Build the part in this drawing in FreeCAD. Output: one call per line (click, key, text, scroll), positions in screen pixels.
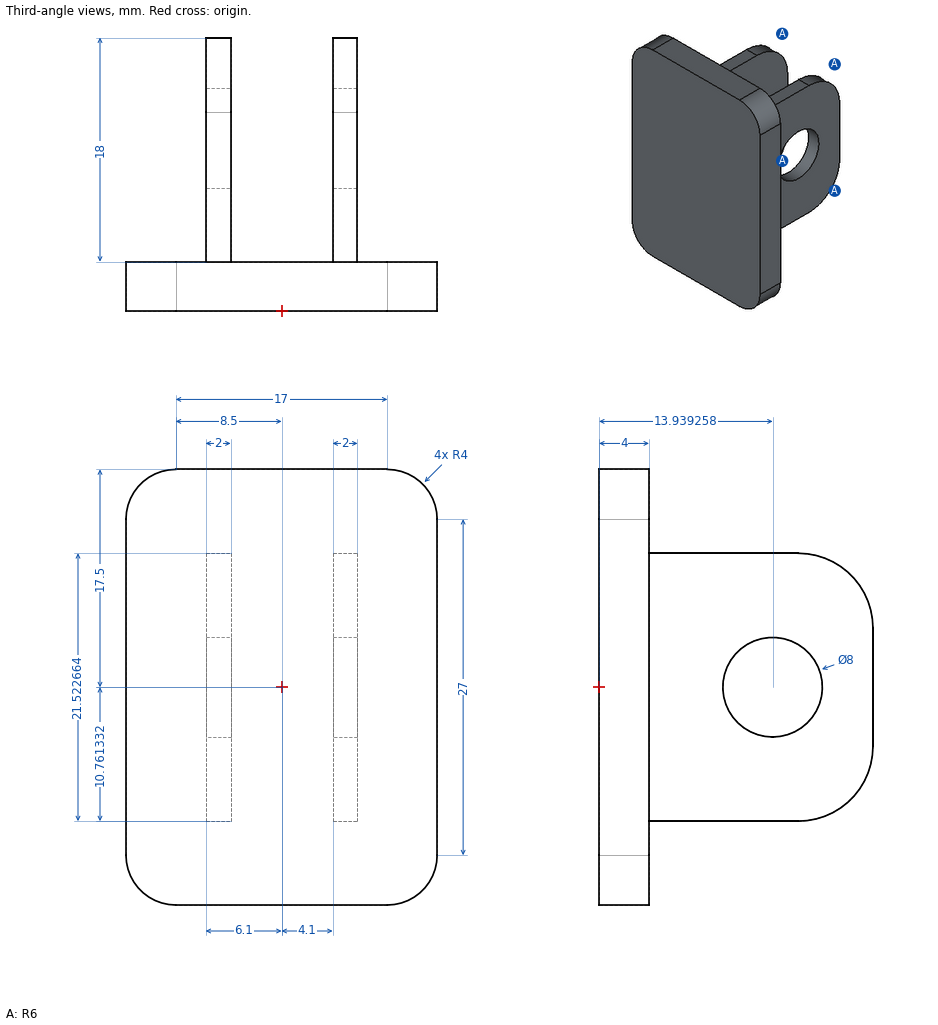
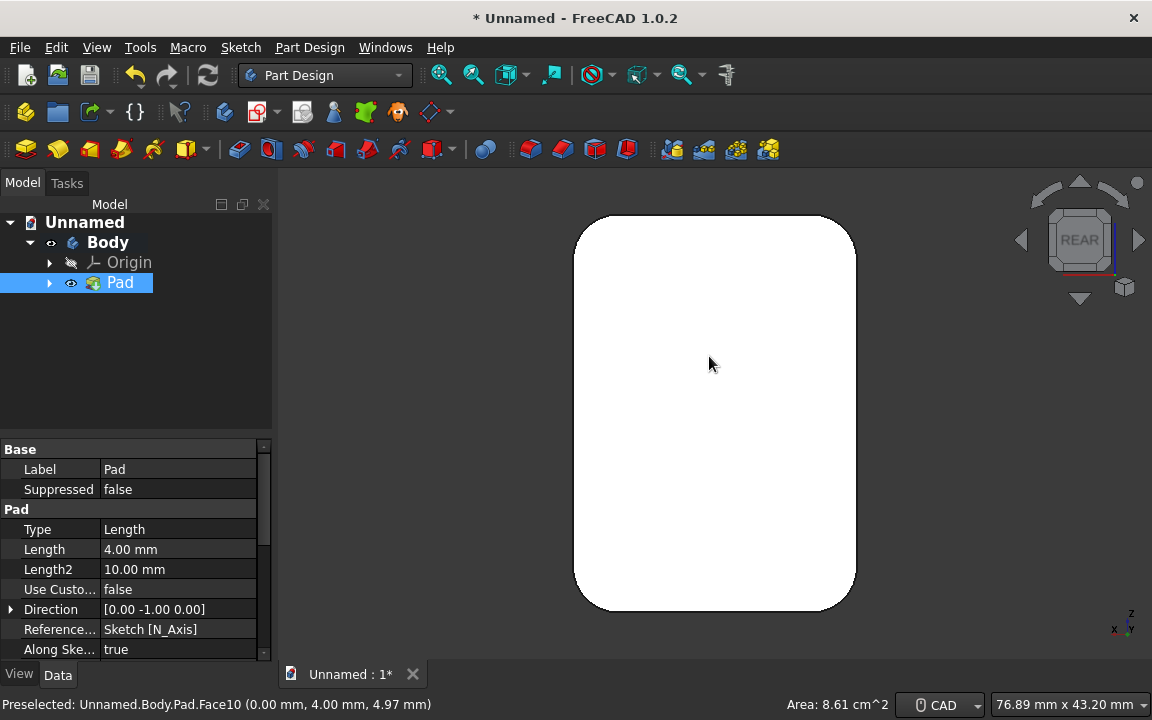
click(258, 112)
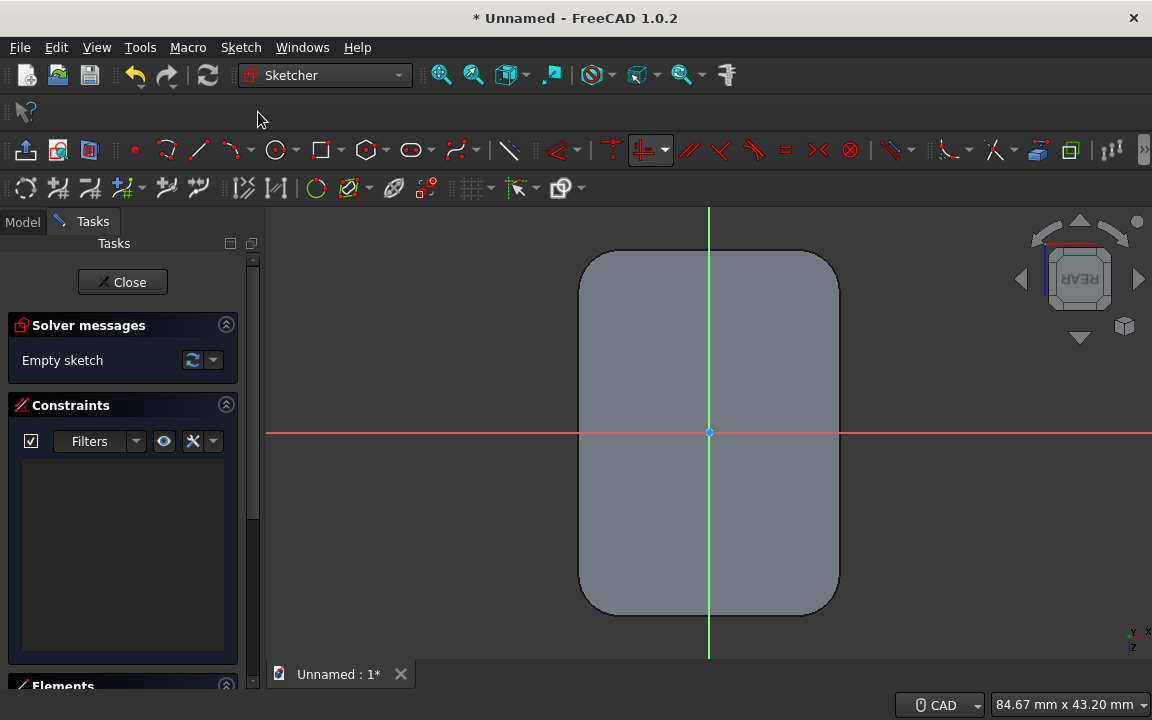
click(322, 150)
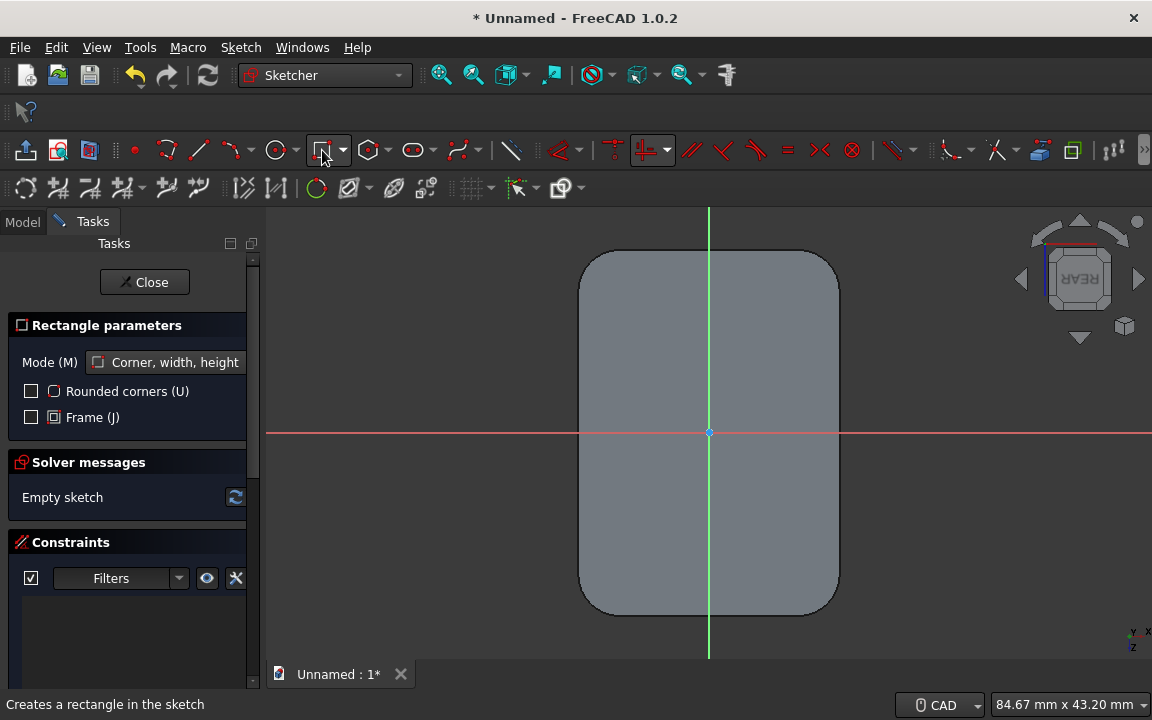
click(645, 320)
move(666, 546)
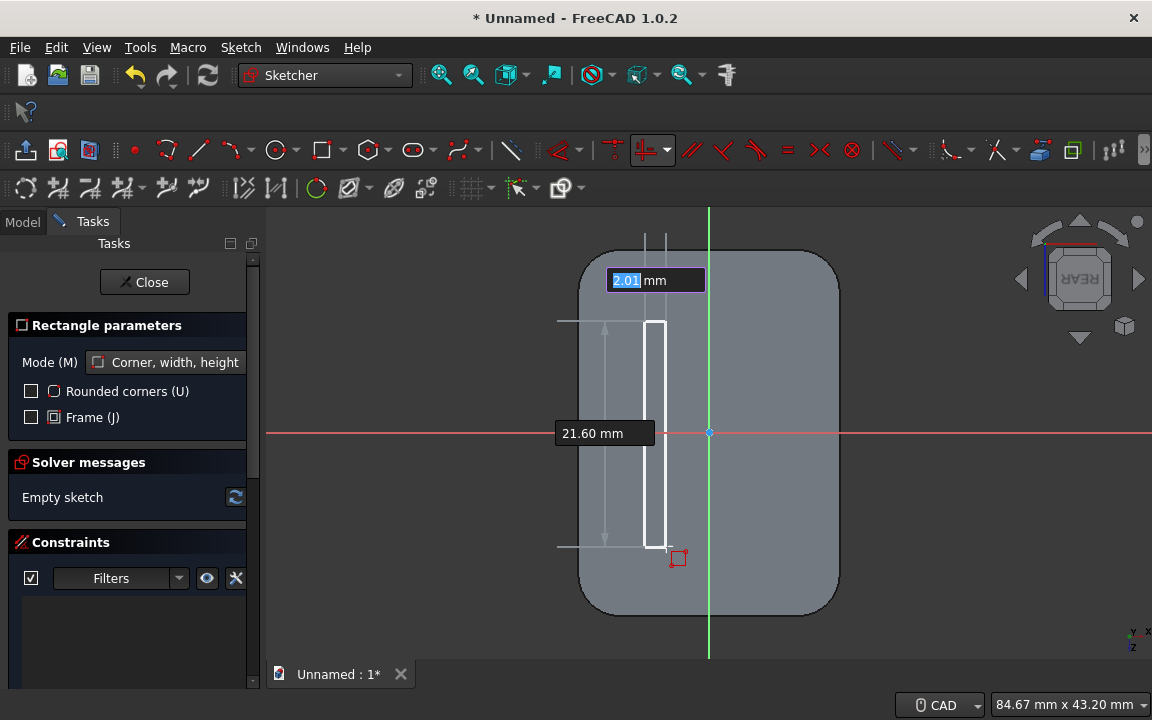
text(2)
key(Tab)
text(21.522664)
key(Return)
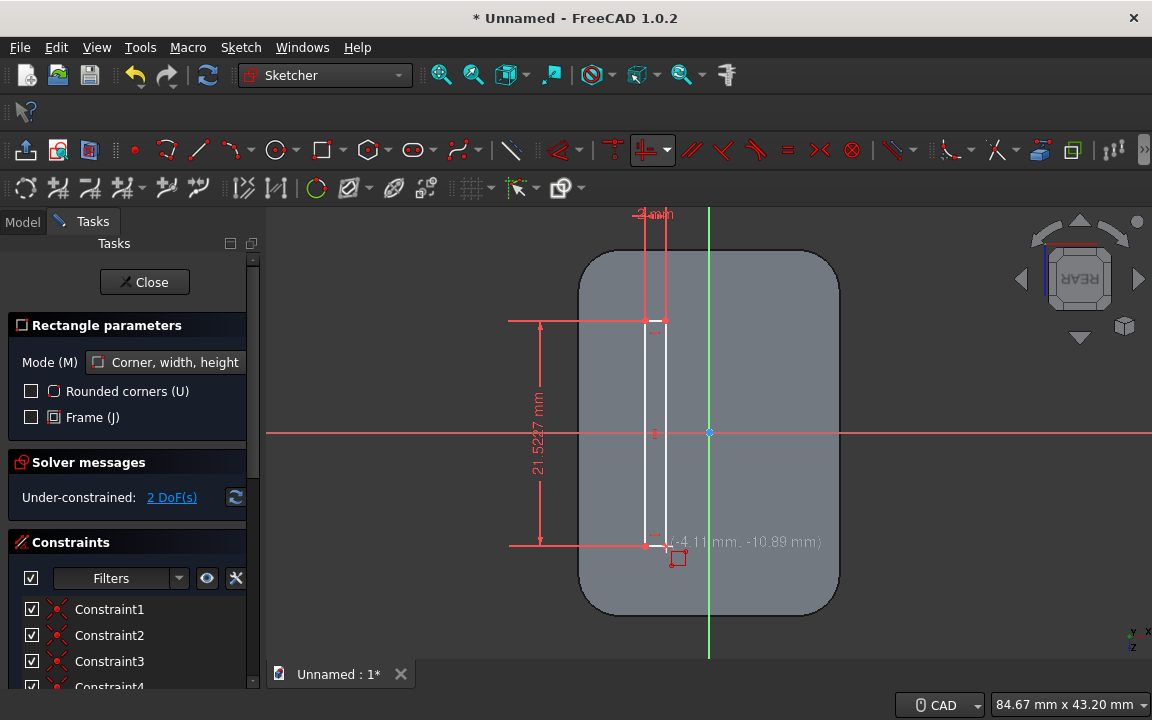
click(752, 320)
move(773, 546)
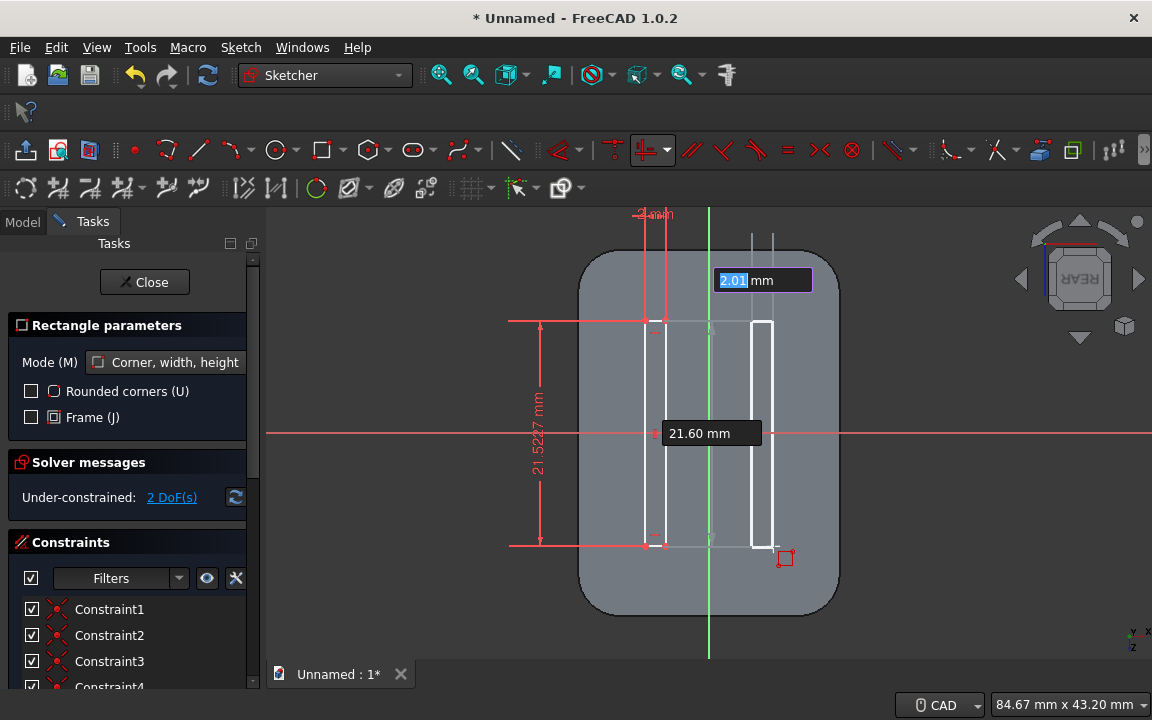
text(2)
key(Tab)
text(21.522664)
key(Return)
key(Escape)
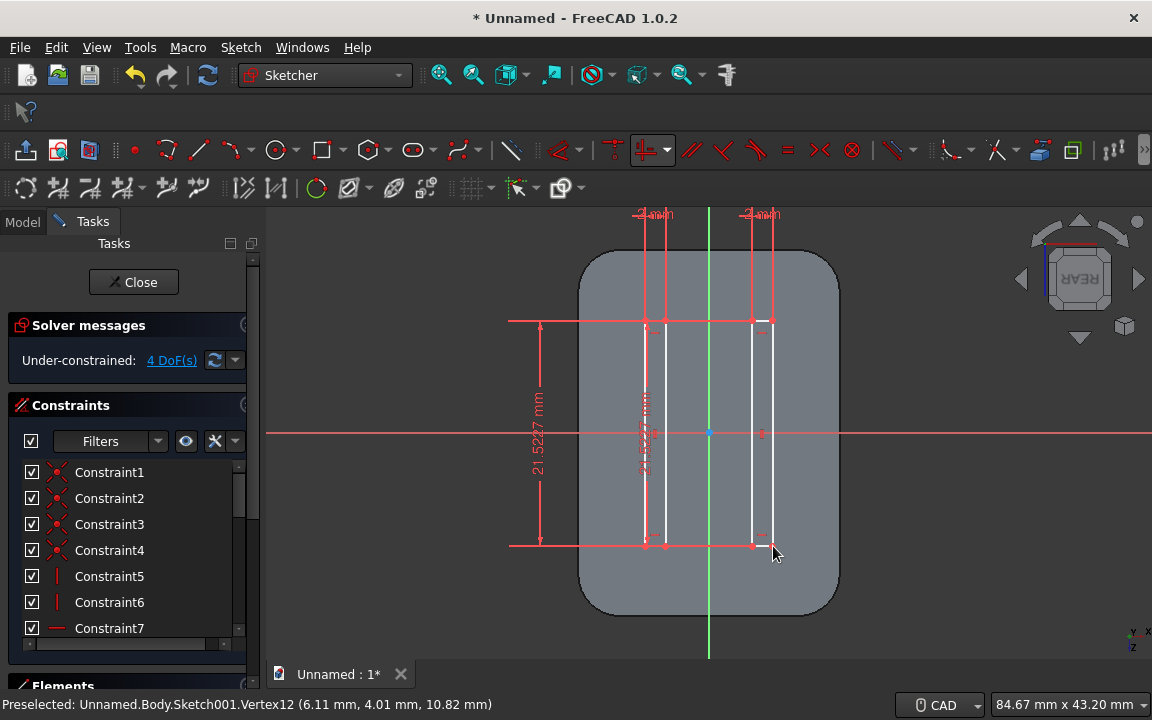
click(558, 150)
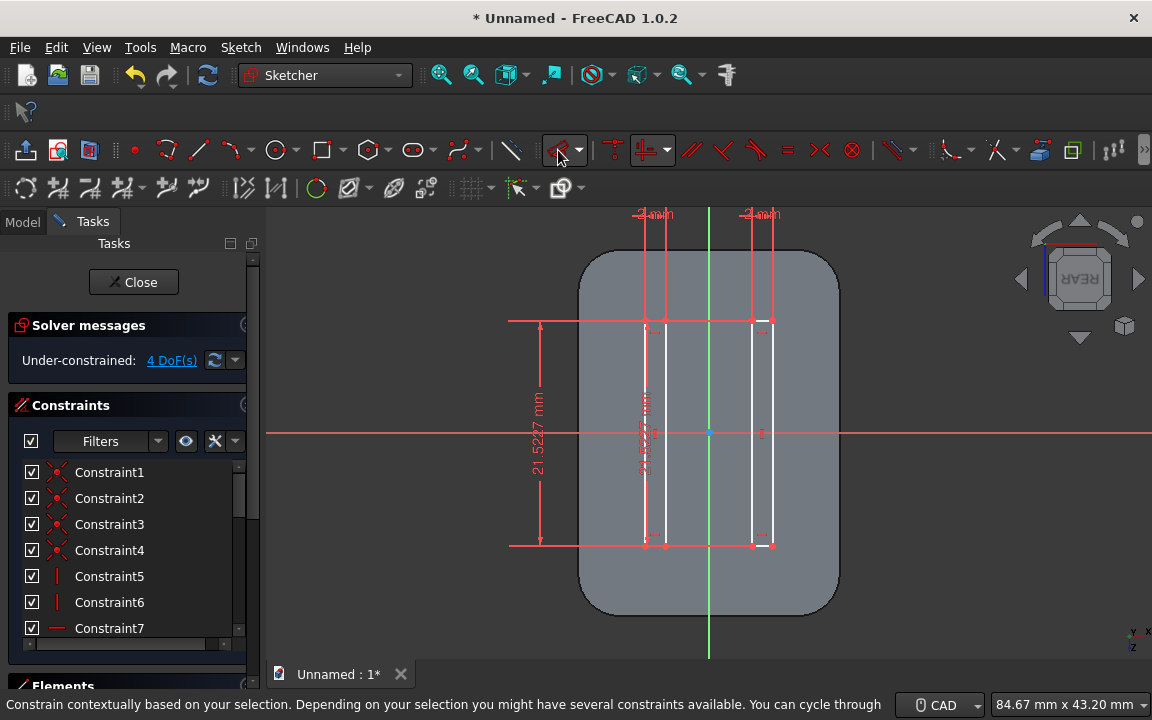
click(645, 321)
click(677, 287)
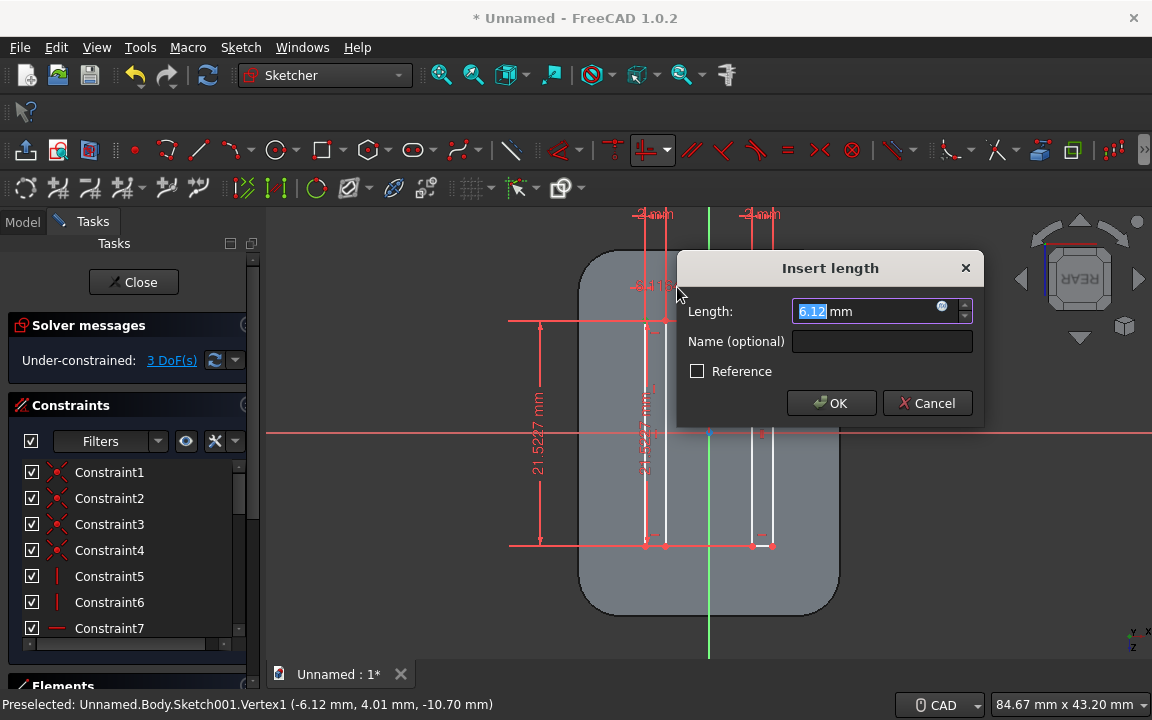
text(6.1)
key(Return)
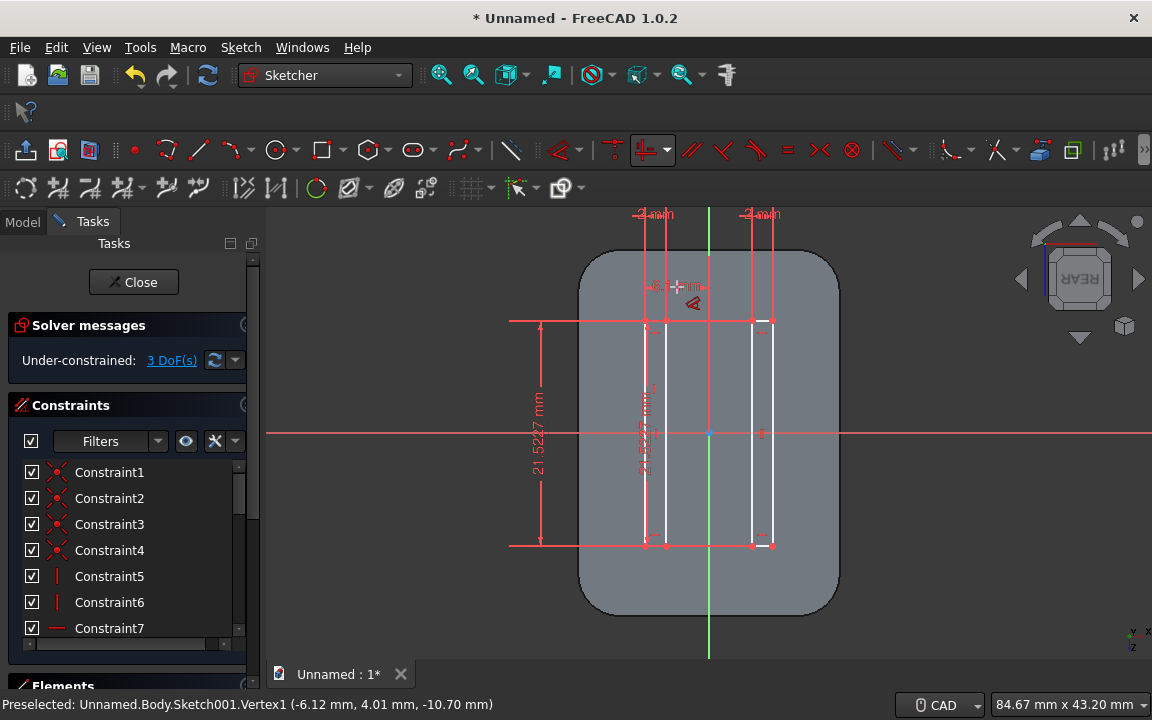
click(752, 321)
click(730, 467)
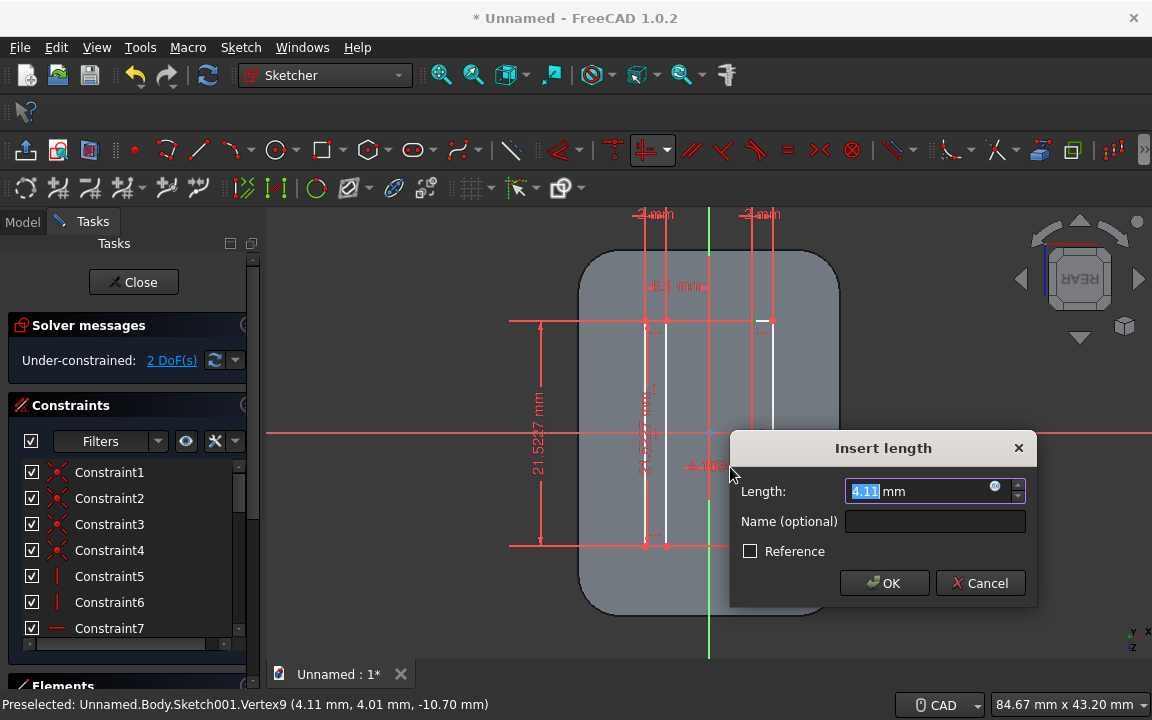
text(4.1)
key(Return)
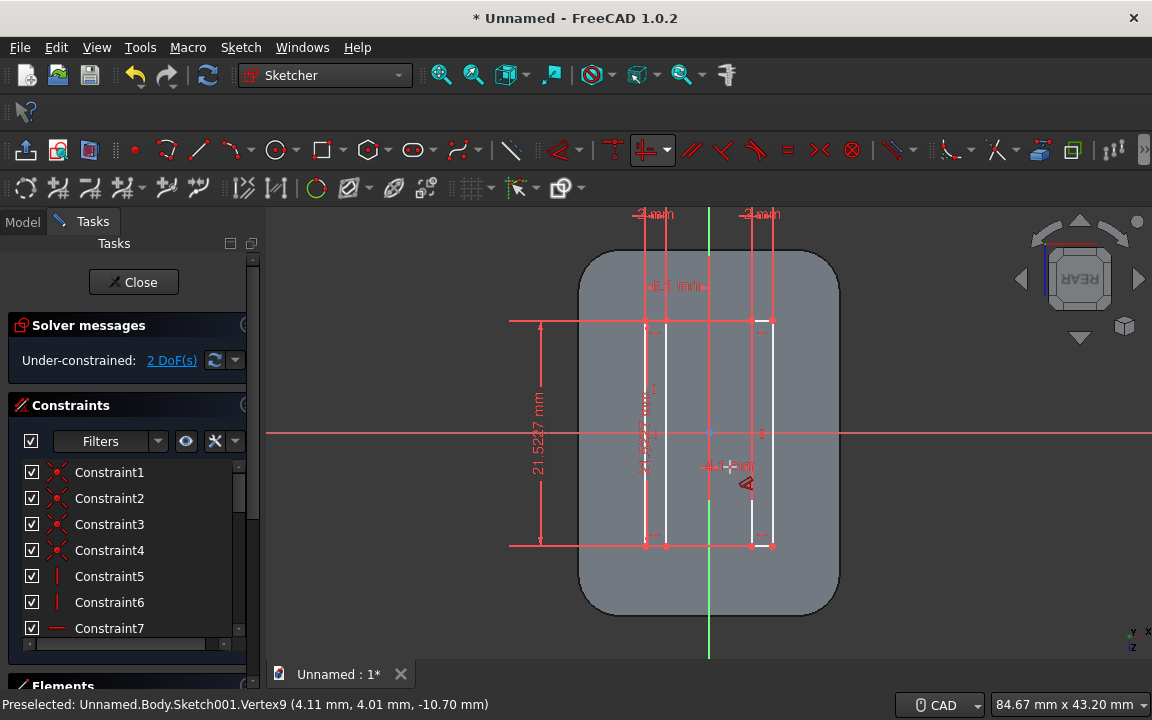
click(645, 321)
click(611, 377)